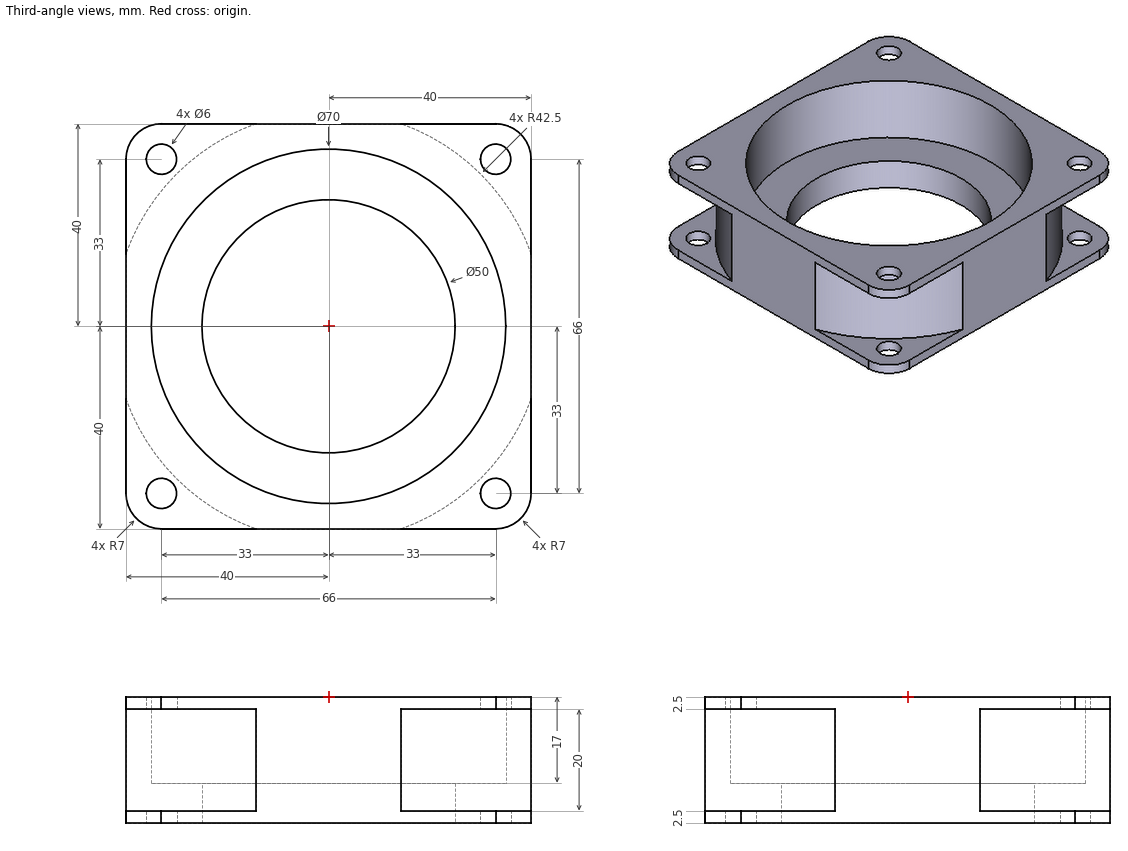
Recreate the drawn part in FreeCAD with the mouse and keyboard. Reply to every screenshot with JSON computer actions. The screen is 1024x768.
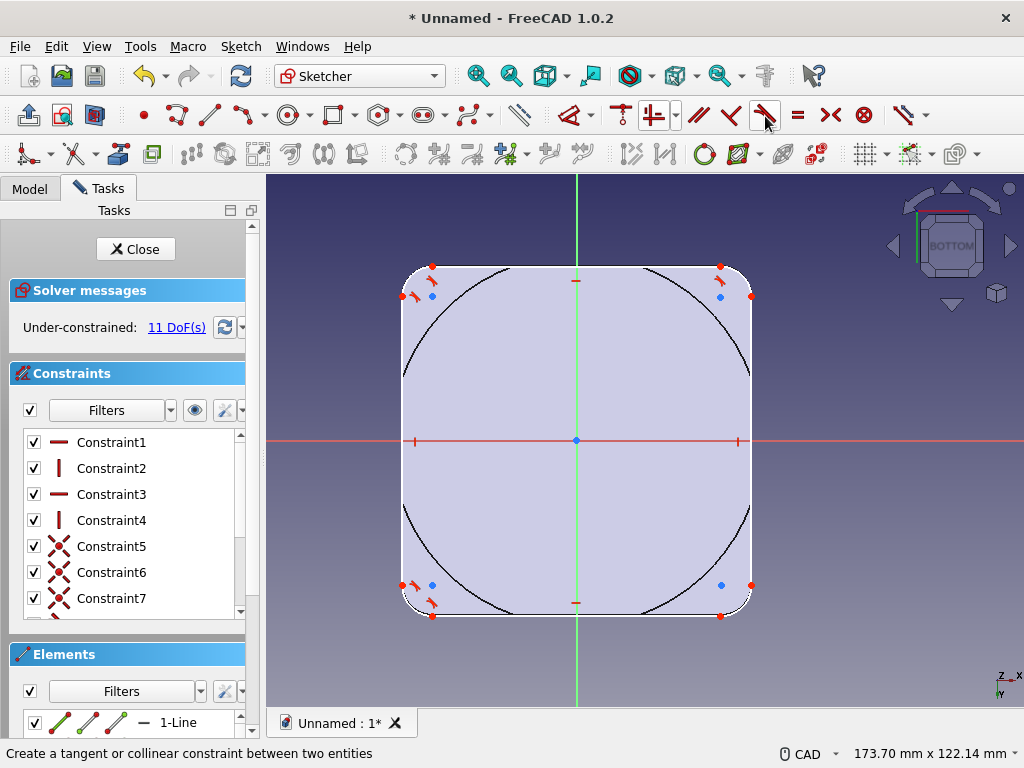
{"action": "left_click", "coordinate": [519, 616]}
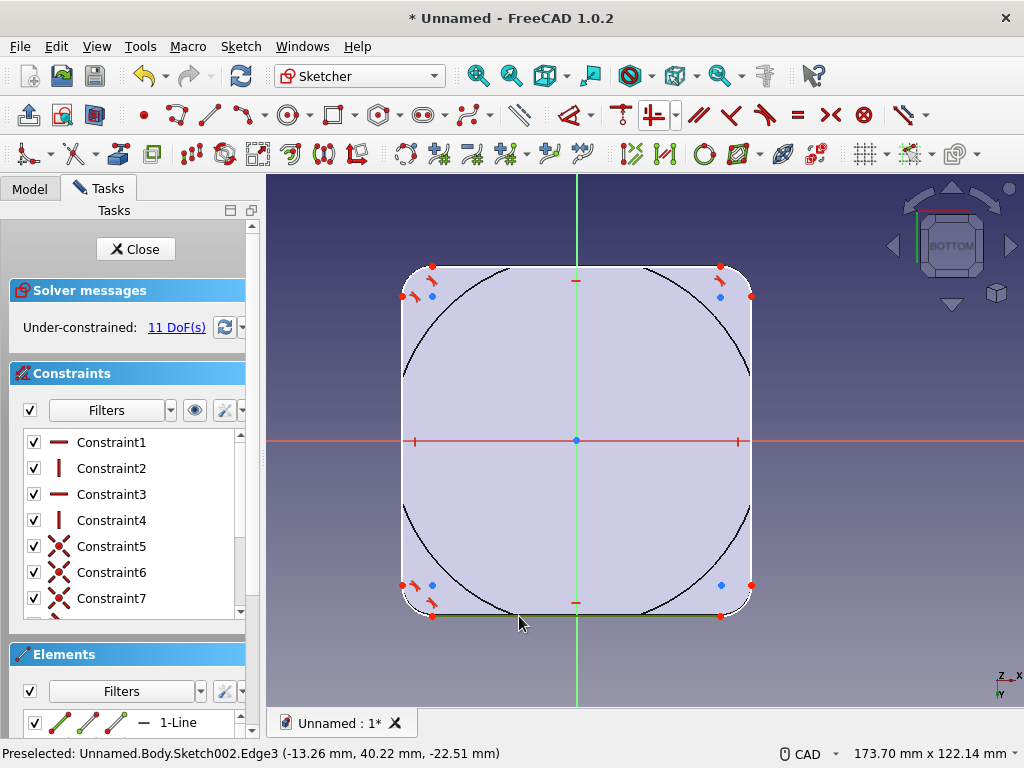
{"action": "left_click", "coordinate": [734, 613]}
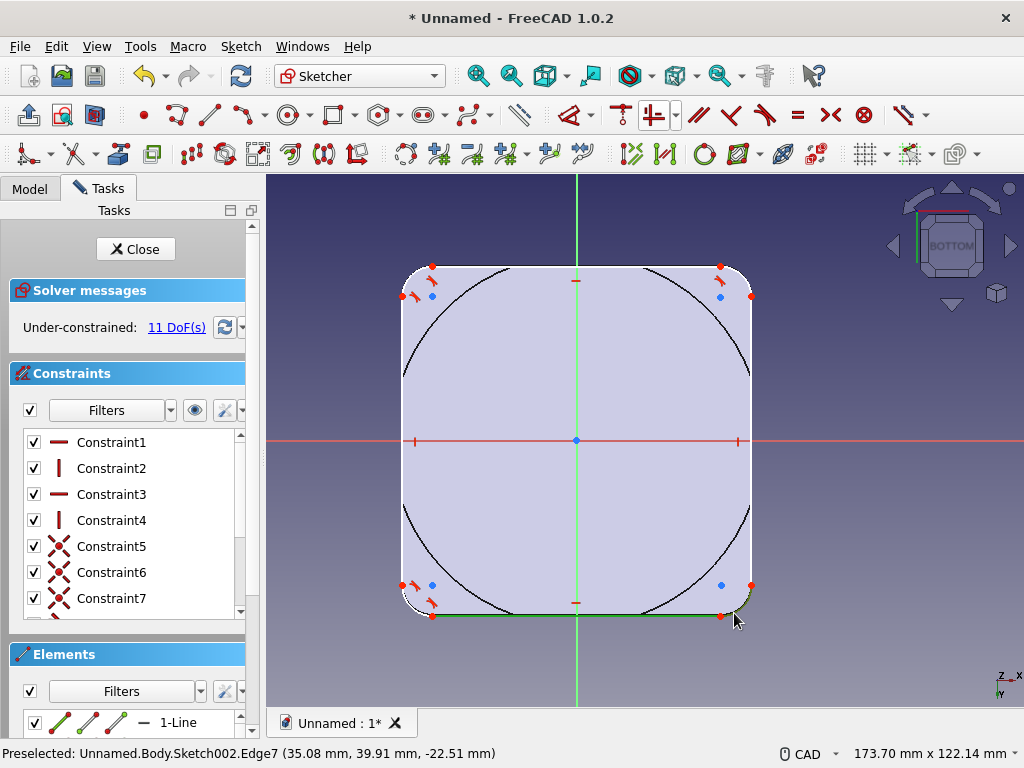
{"action": "left_click", "coordinate": [765, 116]}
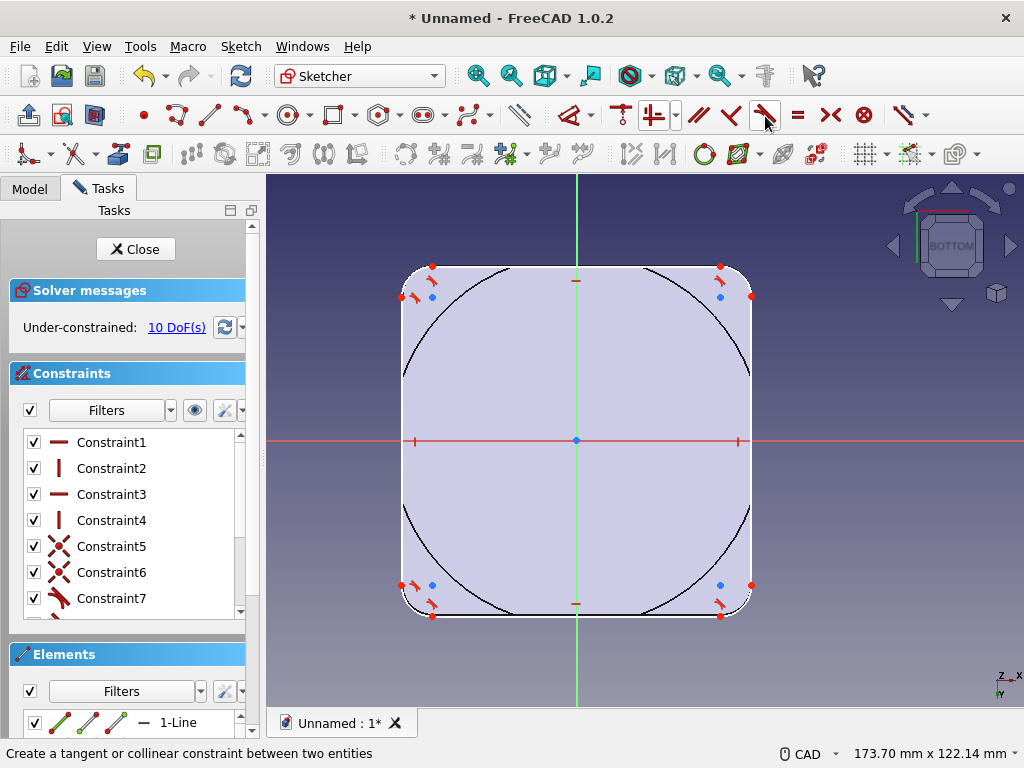
{"action": "left_click", "coordinate": [751, 499]}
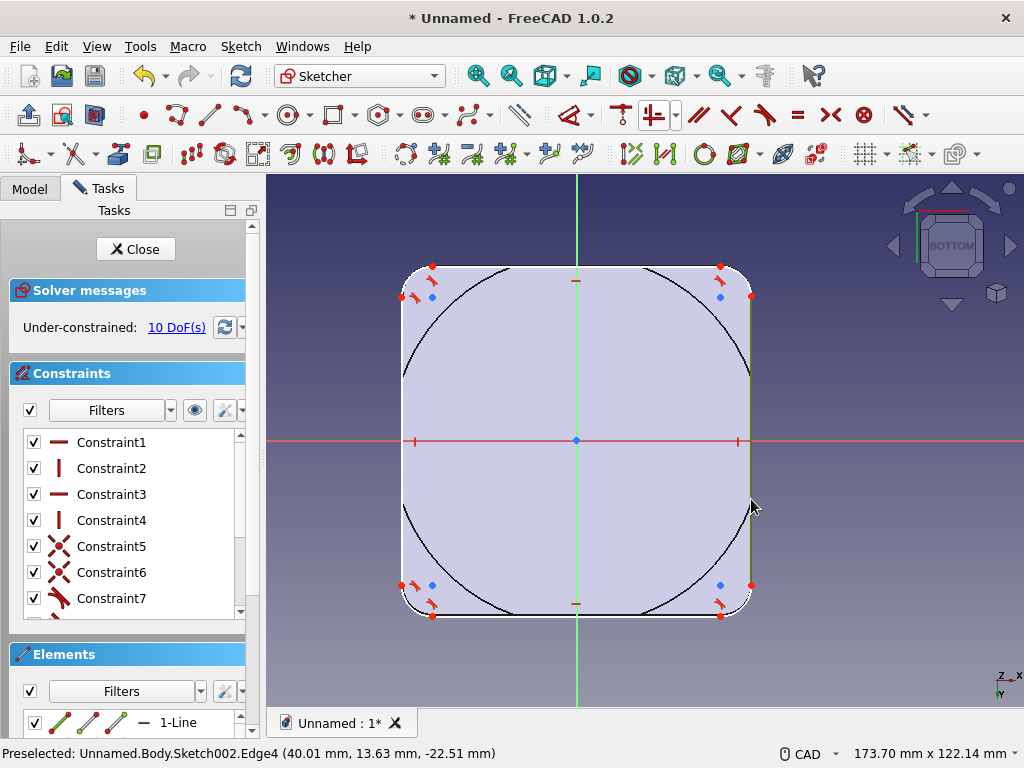
{"action": "left_click", "coordinate": [734, 613]}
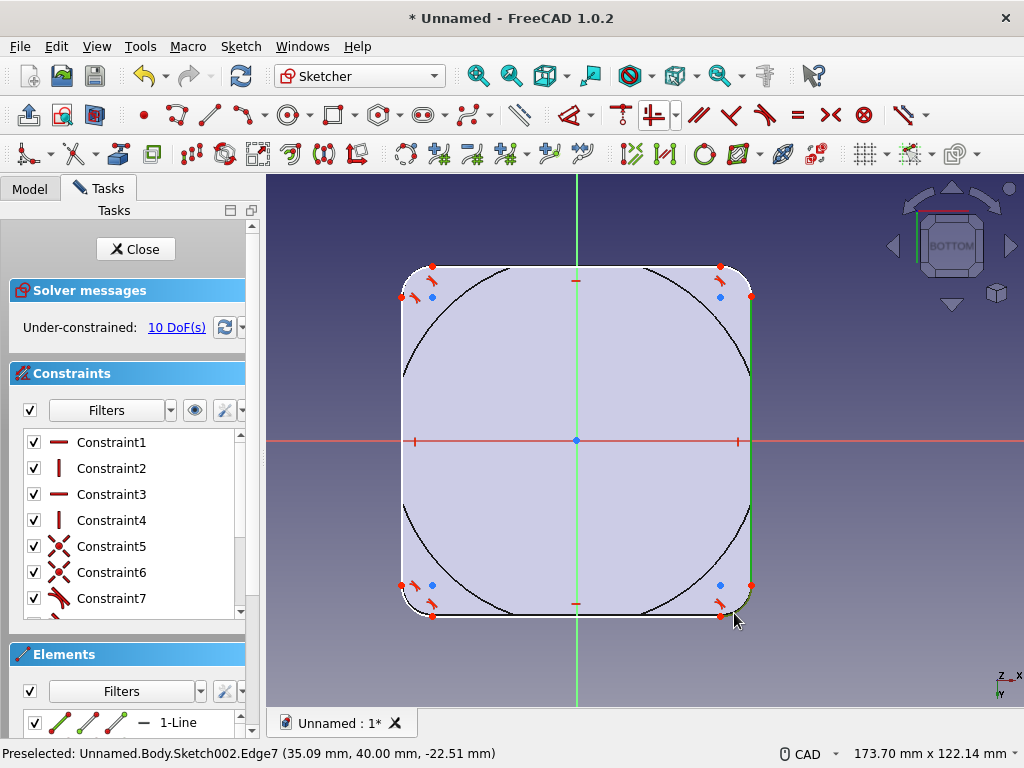
{"action": "left_click", "coordinate": [765, 116]}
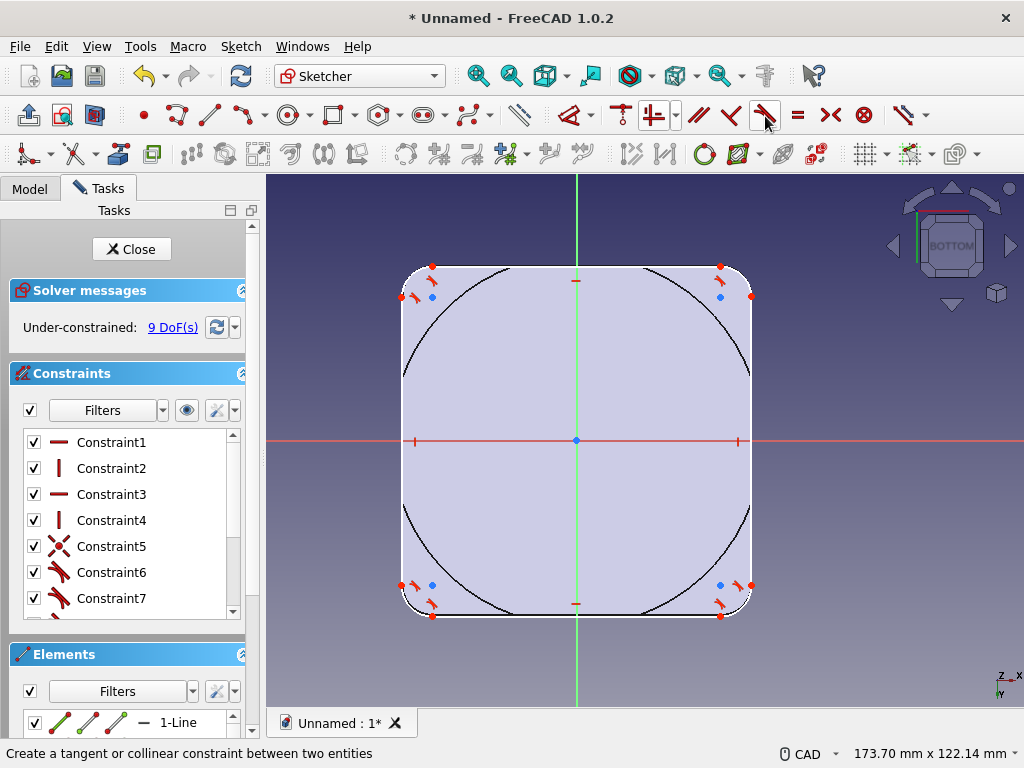
{"action": "left_click", "coordinate": [751, 499]}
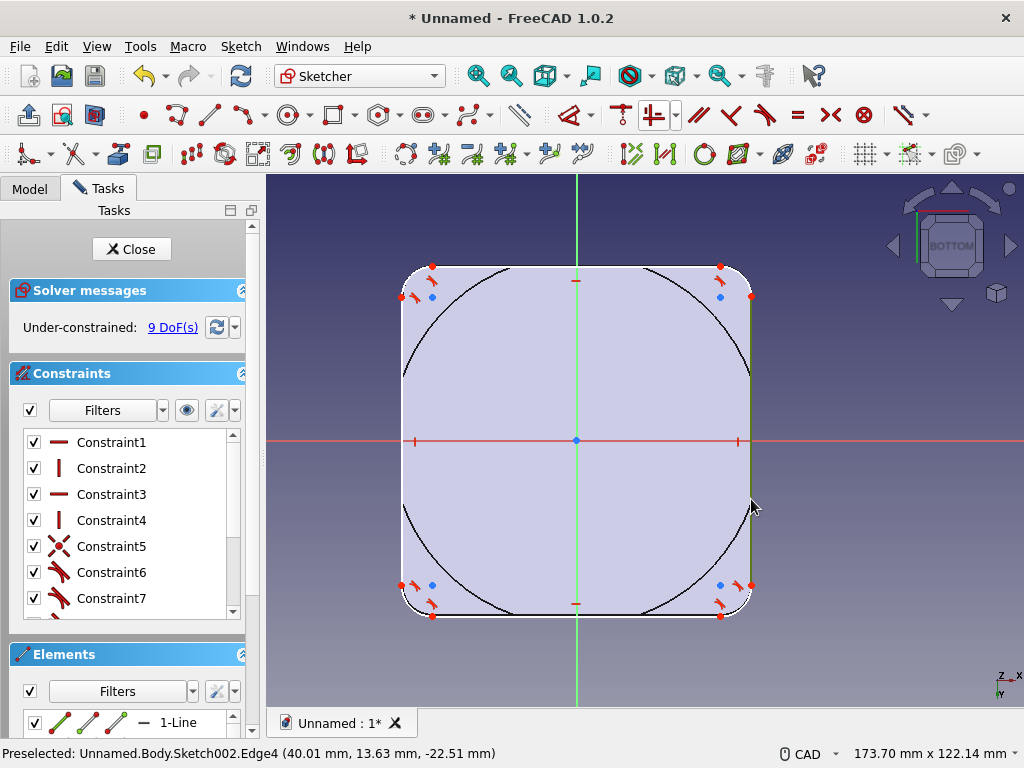
{"action": "left_click", "coordinate": [748, 283]}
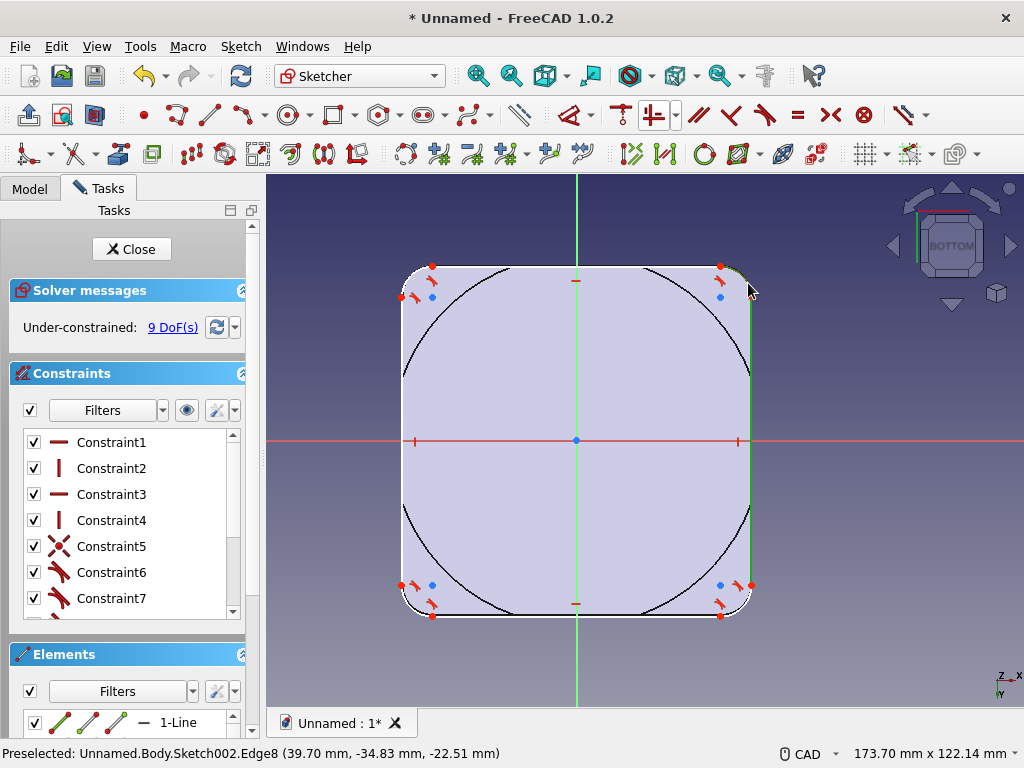
{"action": "left_click", "coordinate": [765, 116]}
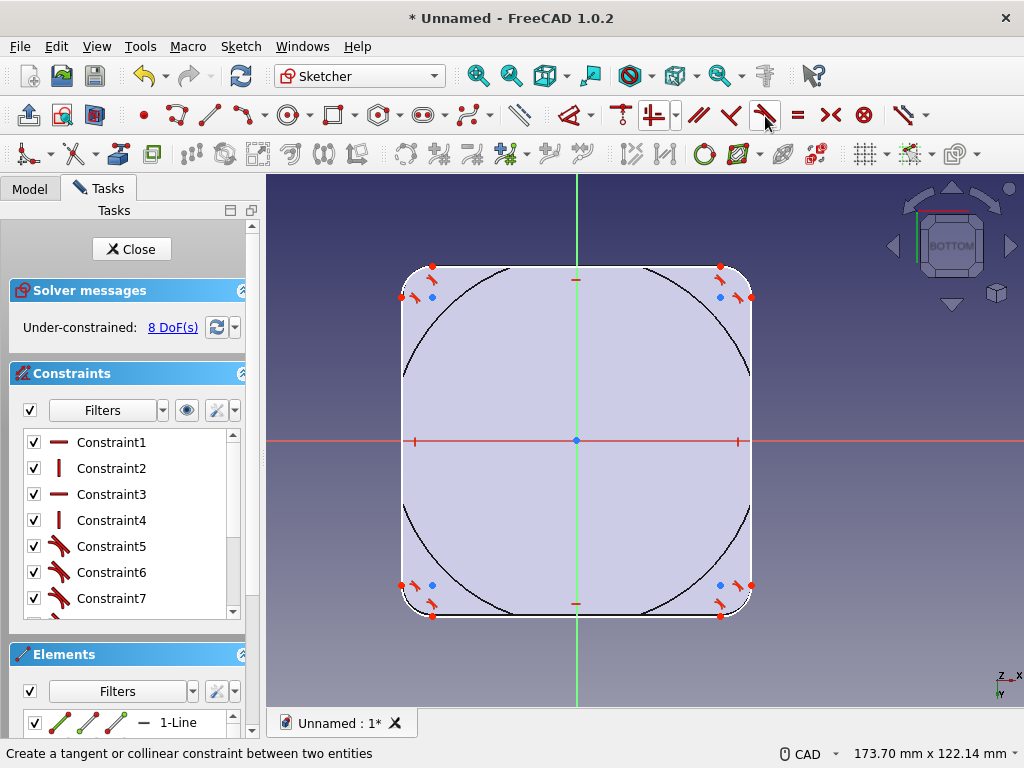
{"action": "left_click", "coordinate": [419, 270]}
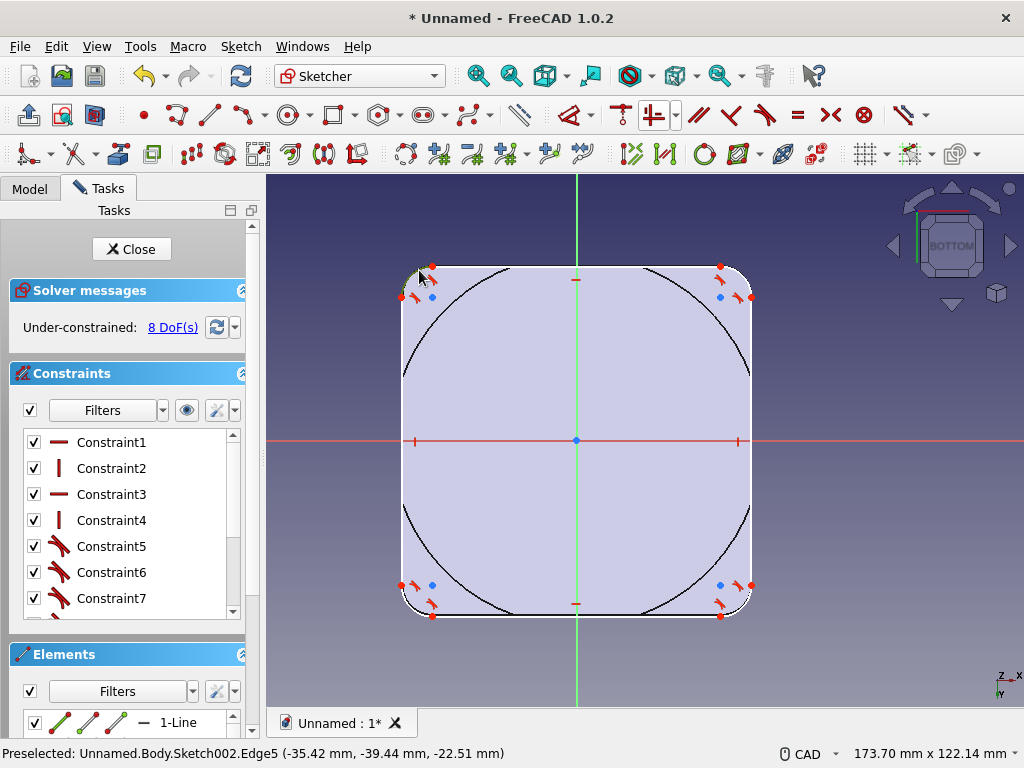
{"action": "left_click", "coordinate": [405, 600]}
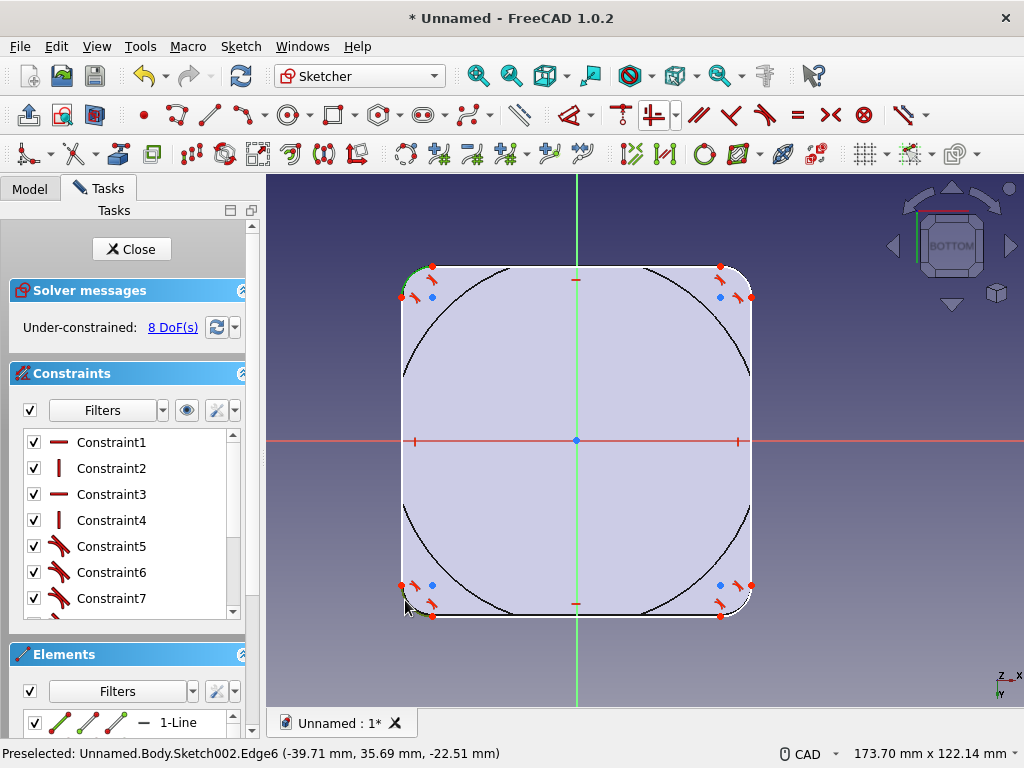
{"action": "left_click", "coordinate": [735, 613]}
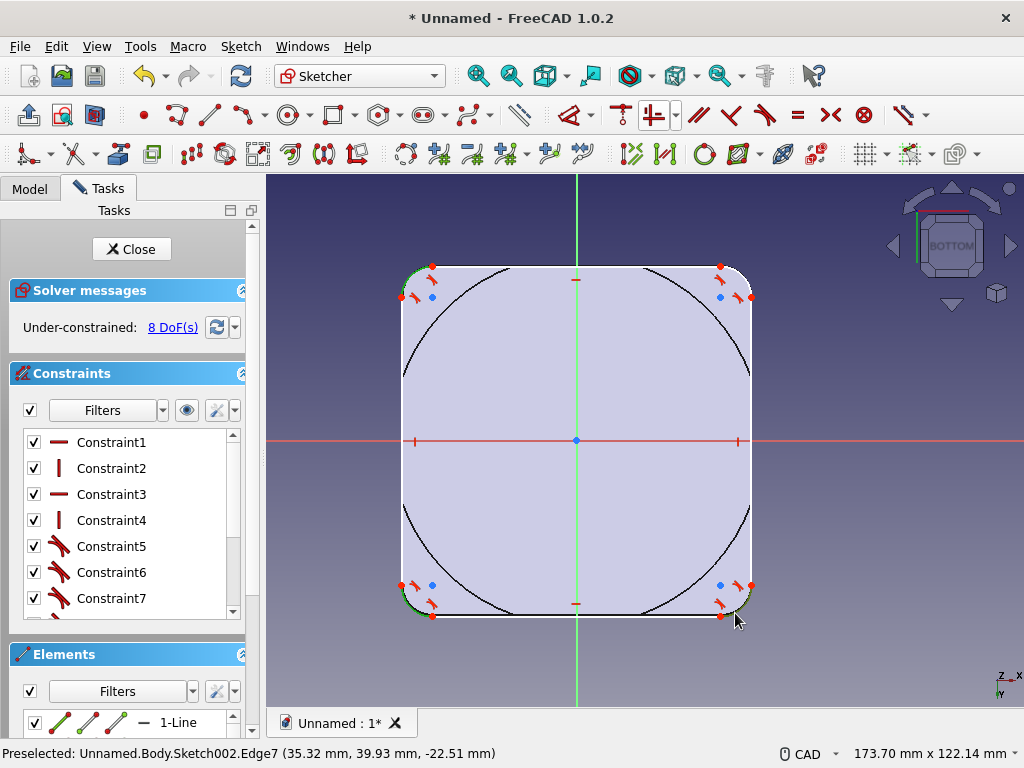
{"action": "left_click", "coordinate": [748, 283]}